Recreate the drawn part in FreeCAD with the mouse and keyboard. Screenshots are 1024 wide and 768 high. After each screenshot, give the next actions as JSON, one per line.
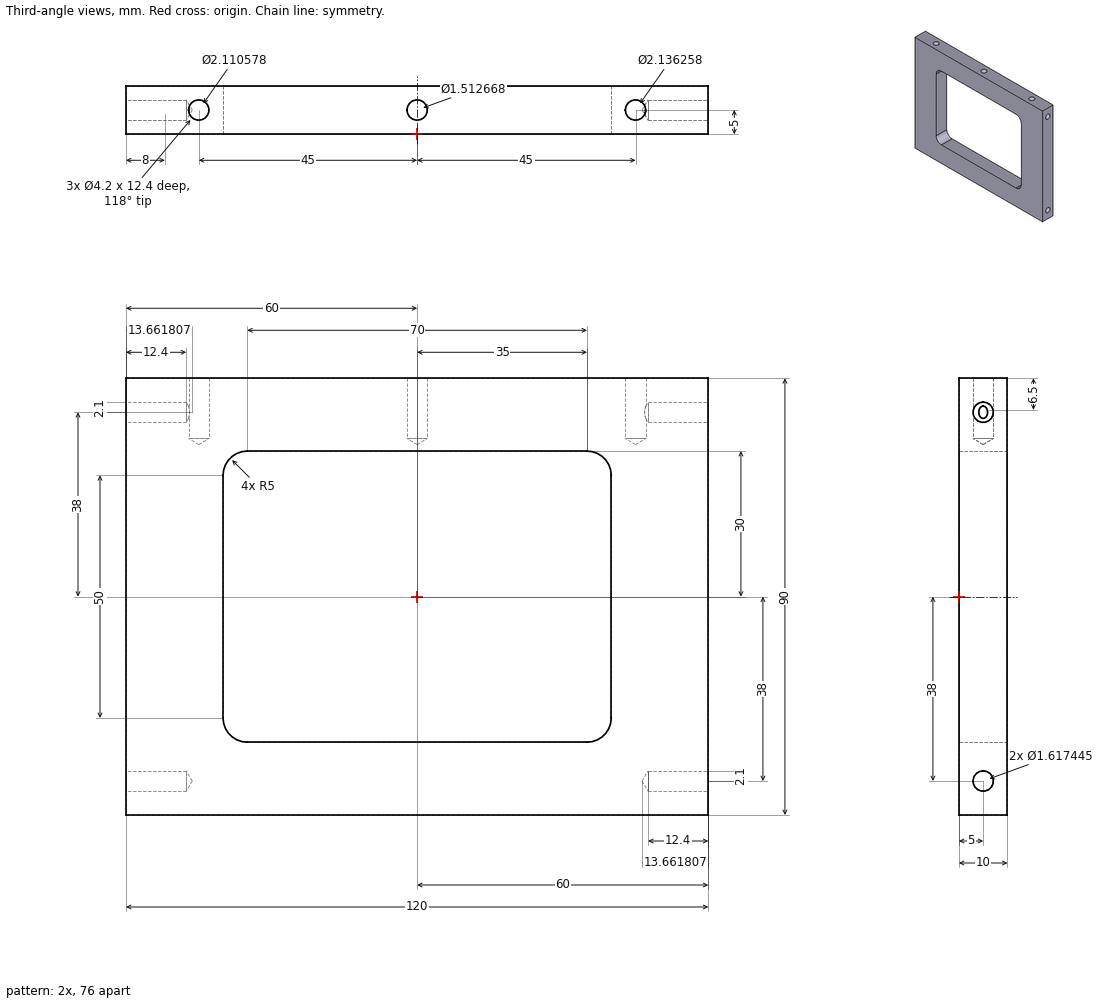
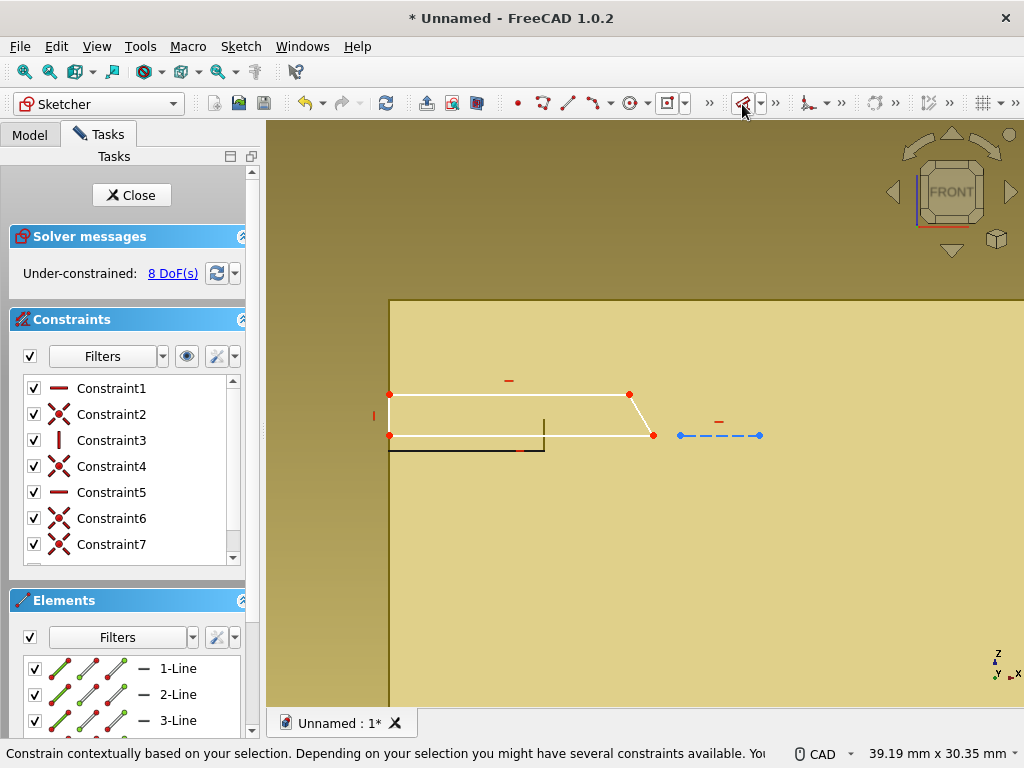
{"action": "left_click", "coordinate": [389, 424]}
{"action": "left_click", "coordinate": [355, 415]}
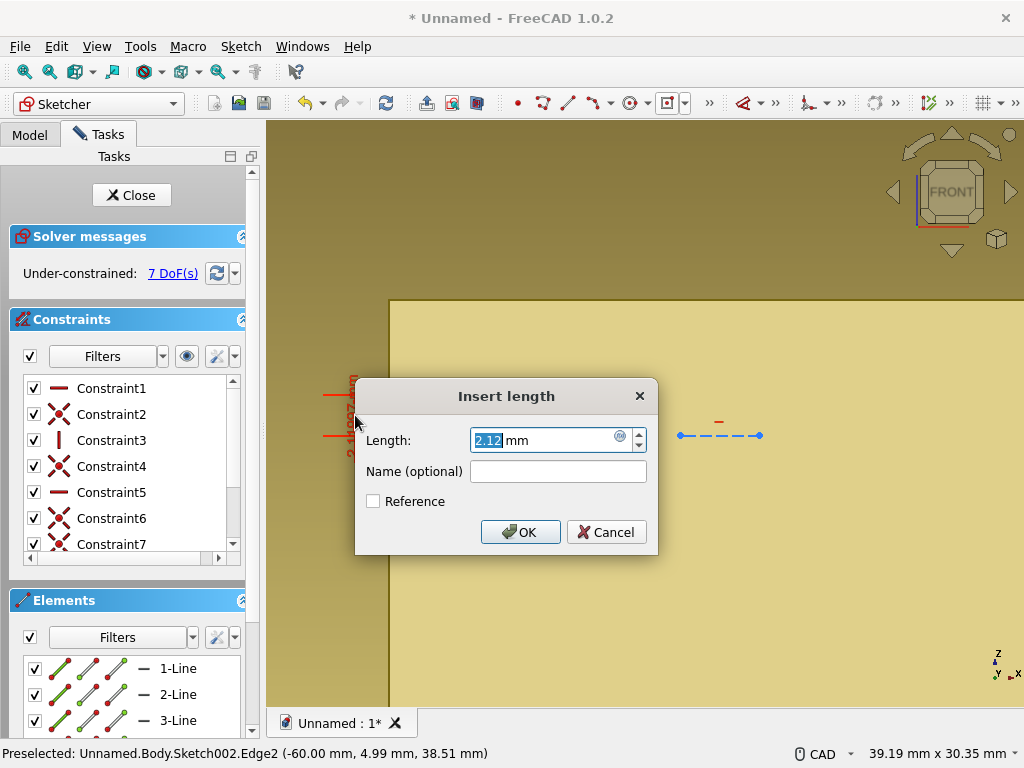
{"action": "type", "text": "2.1"}
{"action": "key", "text": "Return"}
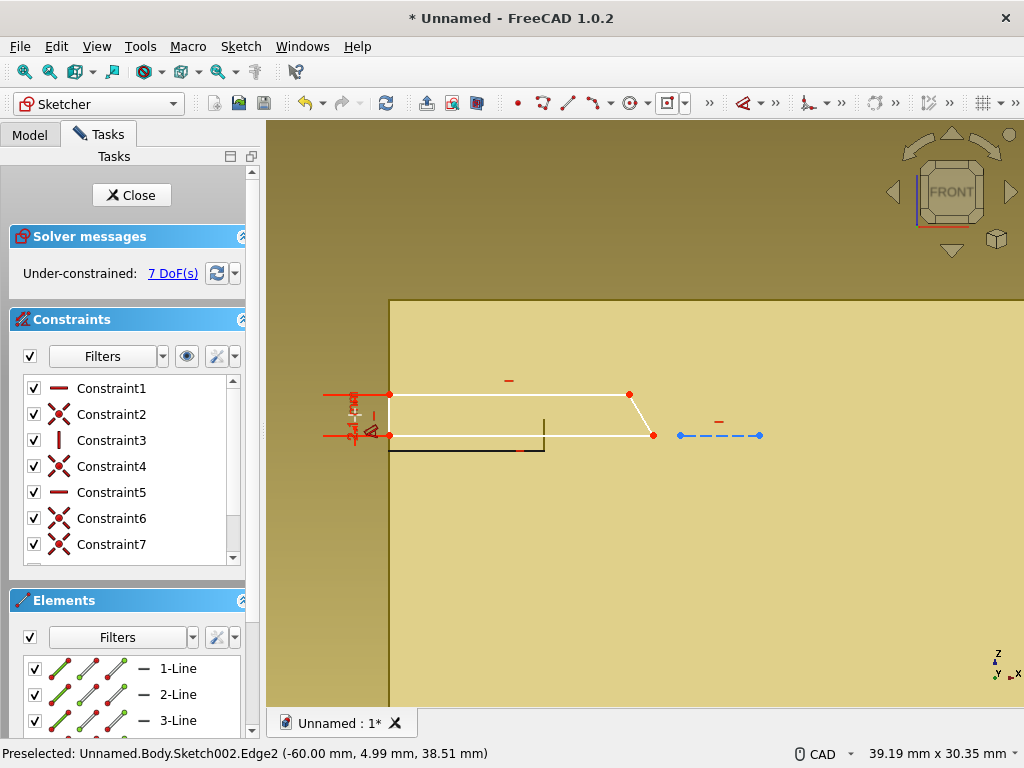
{"action": "left_click", "coordinate": [653, 436]}
{"action": "left_click", "coordinate": [619, 557]}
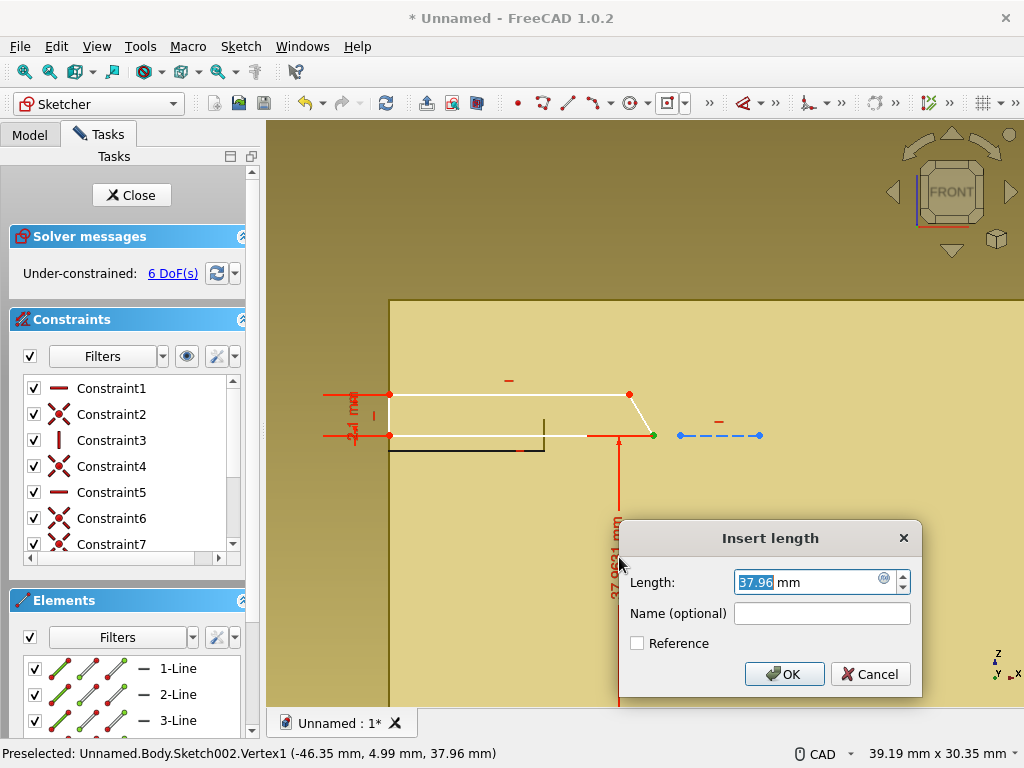
{"action": "type", "text": "38"}
{"action": "key", "text": "Return"}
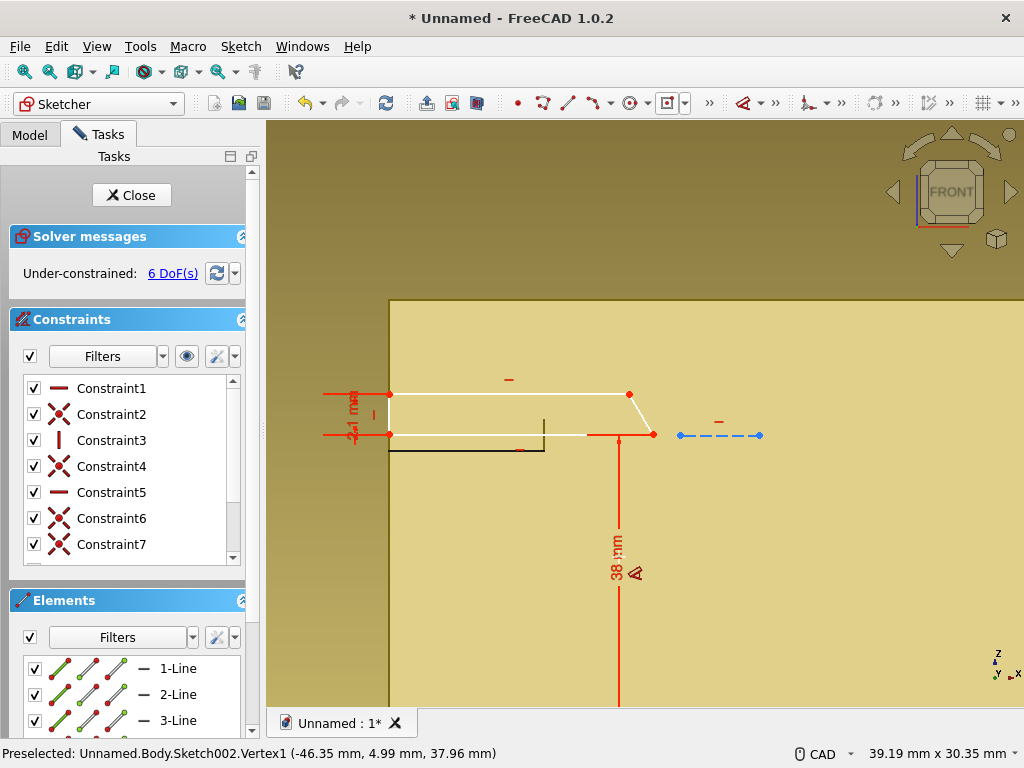
{"action": "left_click", "coordinate": [389, 435]}
{"action": "left_click", "coordinate": [732, 401]}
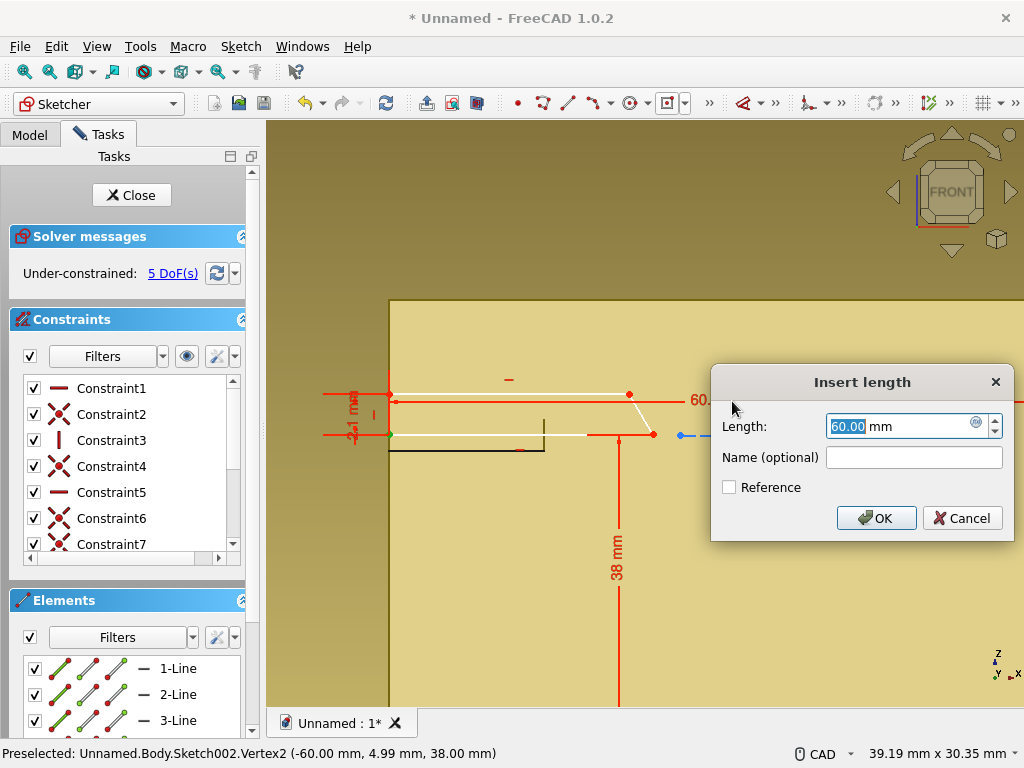
{"action": "type", "text": "60"}
{"action": "key", "text": "Return"}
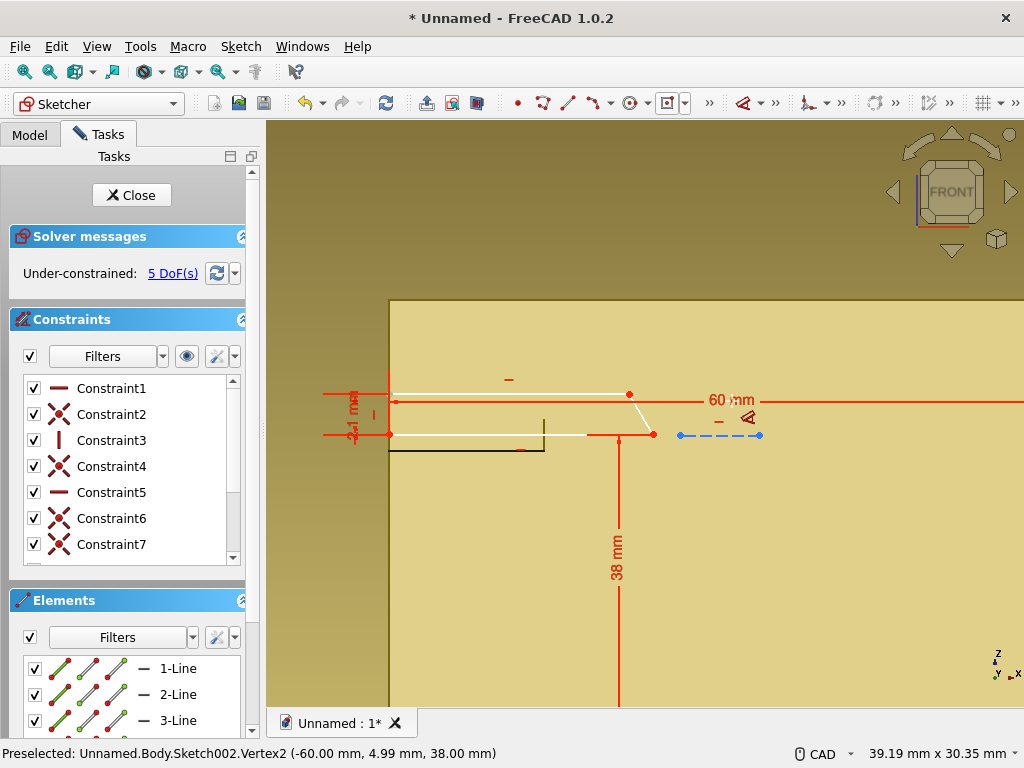
{"action": "left_click", "coordinate": [680, 436]}
{"action": "left_click", "coordinate": [646, 502]}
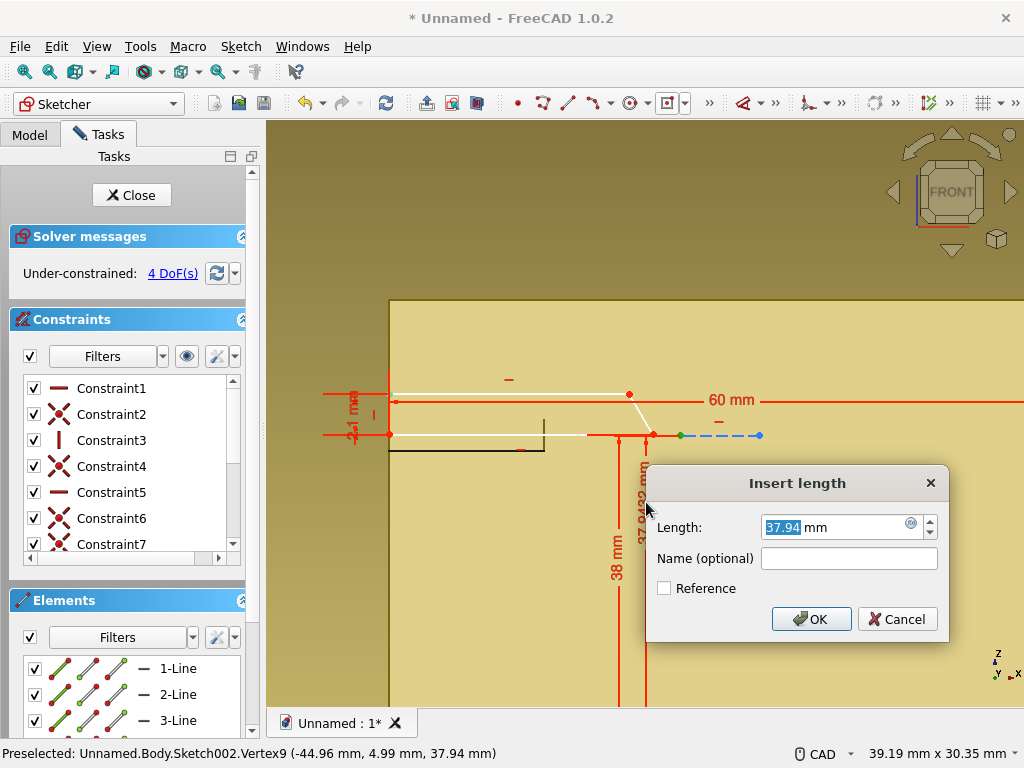
{"action": "type", "text": "38"}
{"action": "key", "text": "Return"}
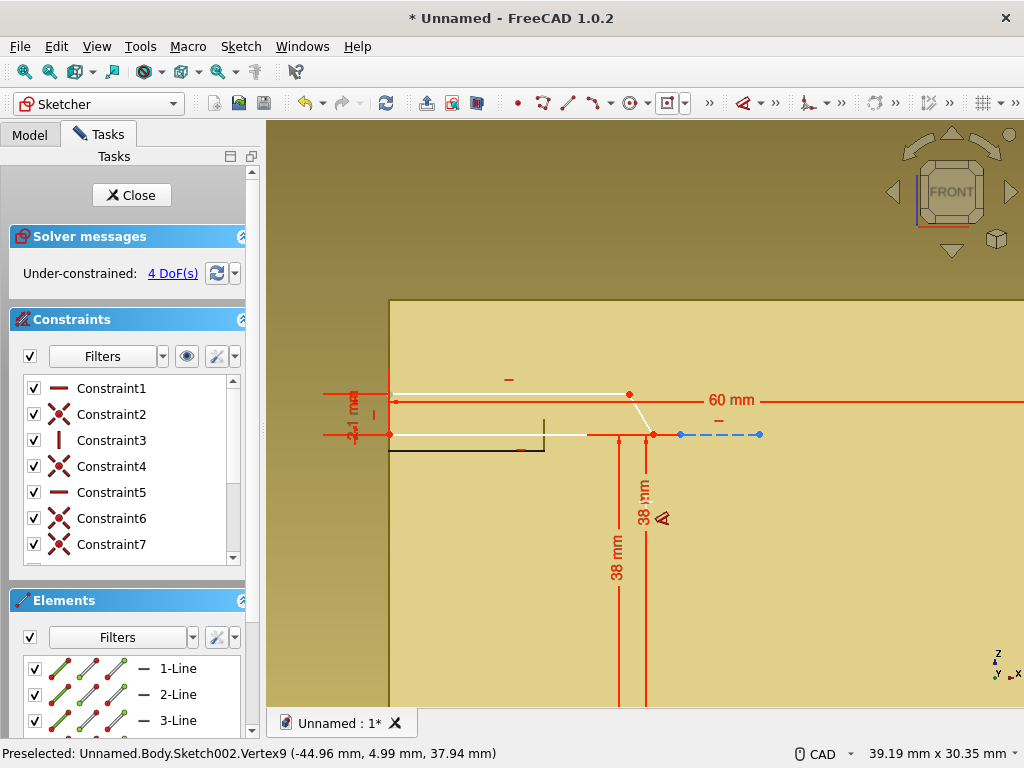
{"action": "left_click", "coordinate": [461, 394]}
{"action": "left_click", "coordinate": [509, 360]}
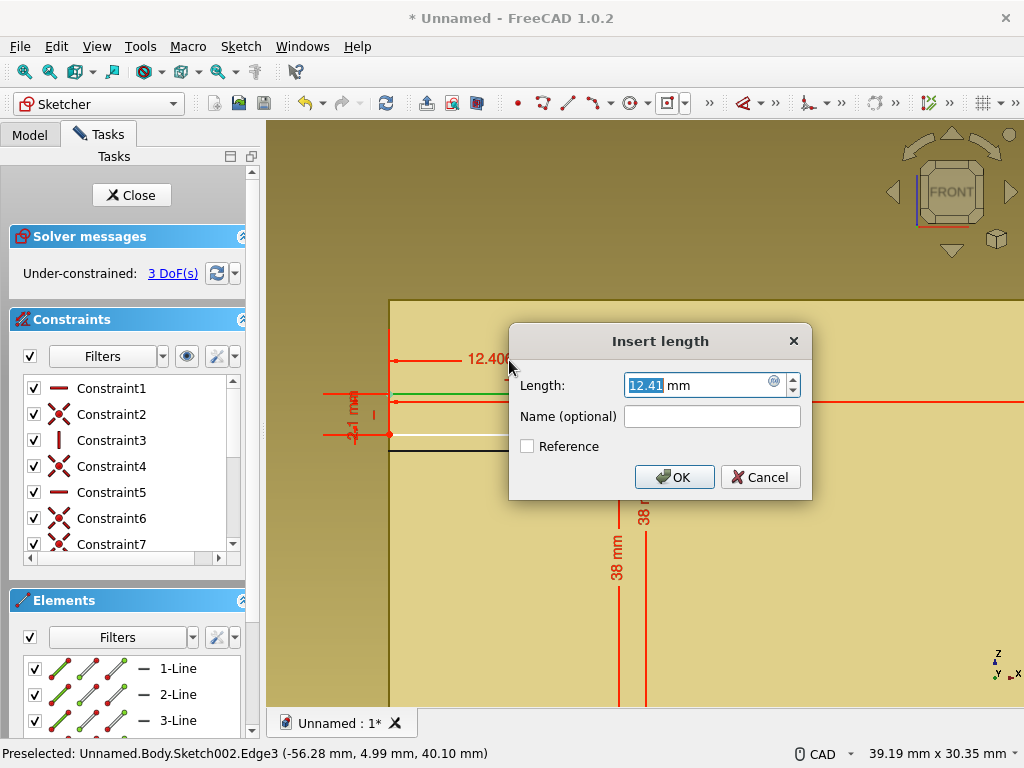
{"action": "type", "text": "12.4"}
{"action": "key", "text": "Return"}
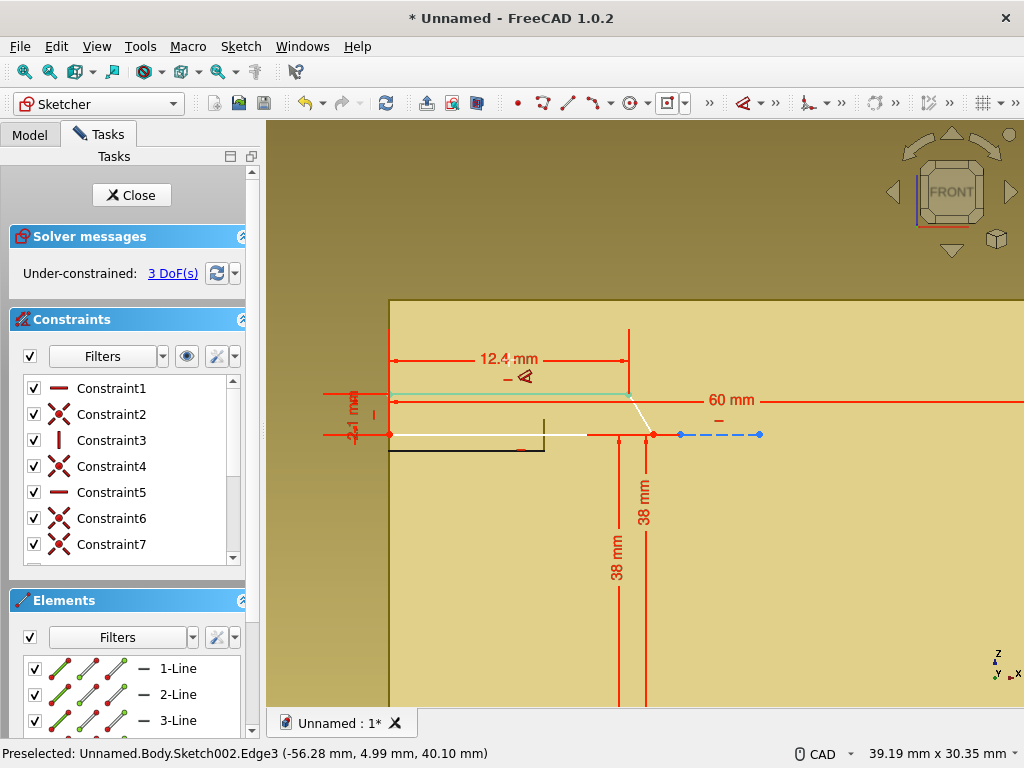
{"action": "left_click", "coordinate": [574, 435]}
{"action": "left_click", "coordinate": [521, 469]}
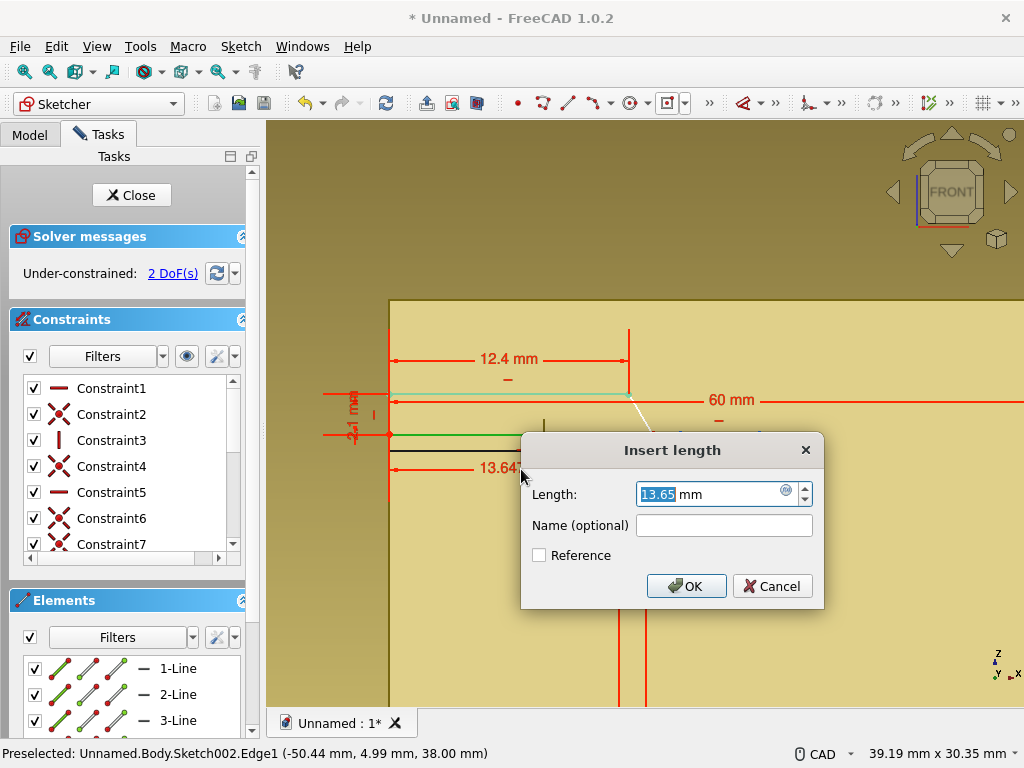
{"action": "type", "text": "13.661807"}
{"action": "key", "text": "Return"}
{"action": "key", "text": "Escape"}